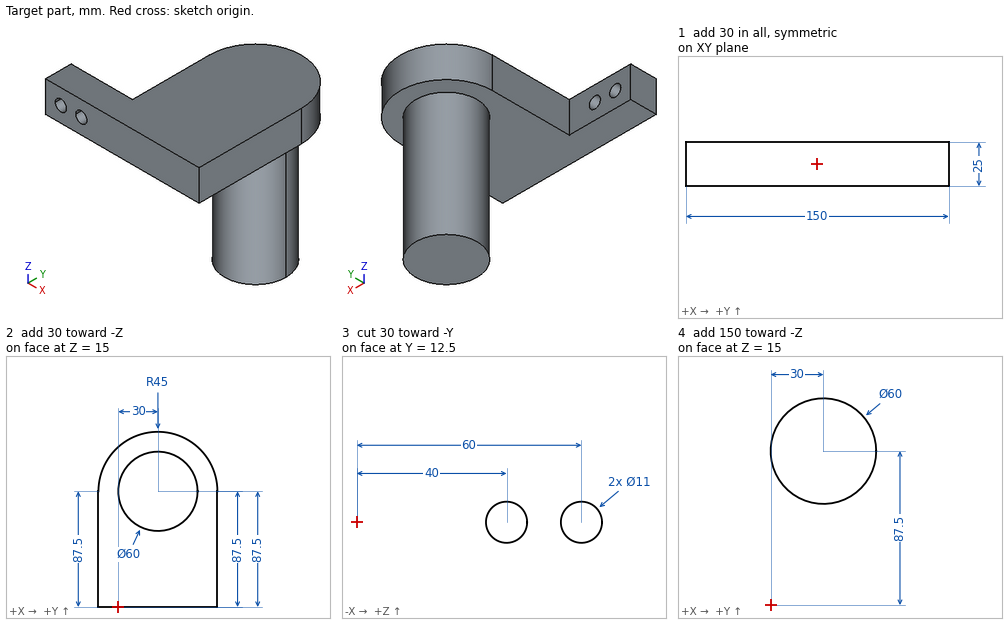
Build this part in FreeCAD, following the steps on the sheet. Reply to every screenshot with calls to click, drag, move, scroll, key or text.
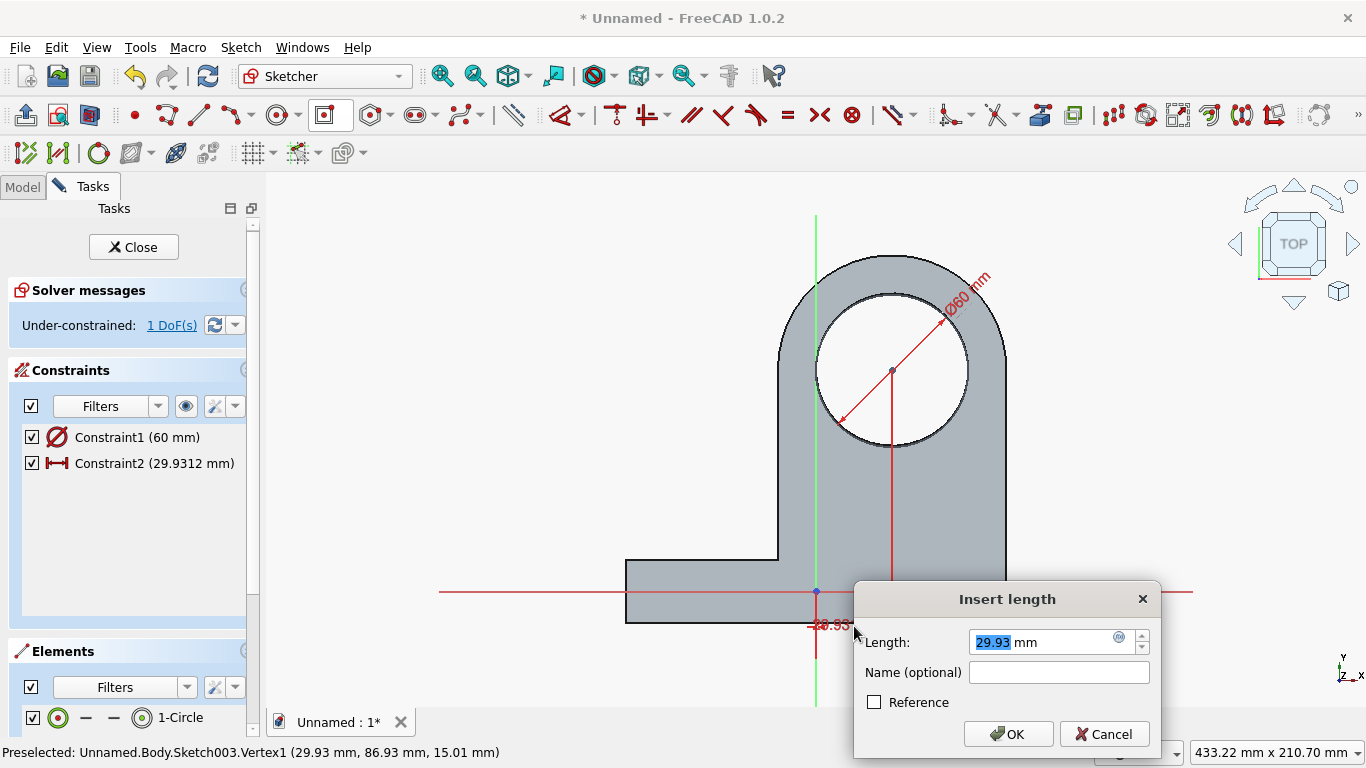
text(30)
key(Return)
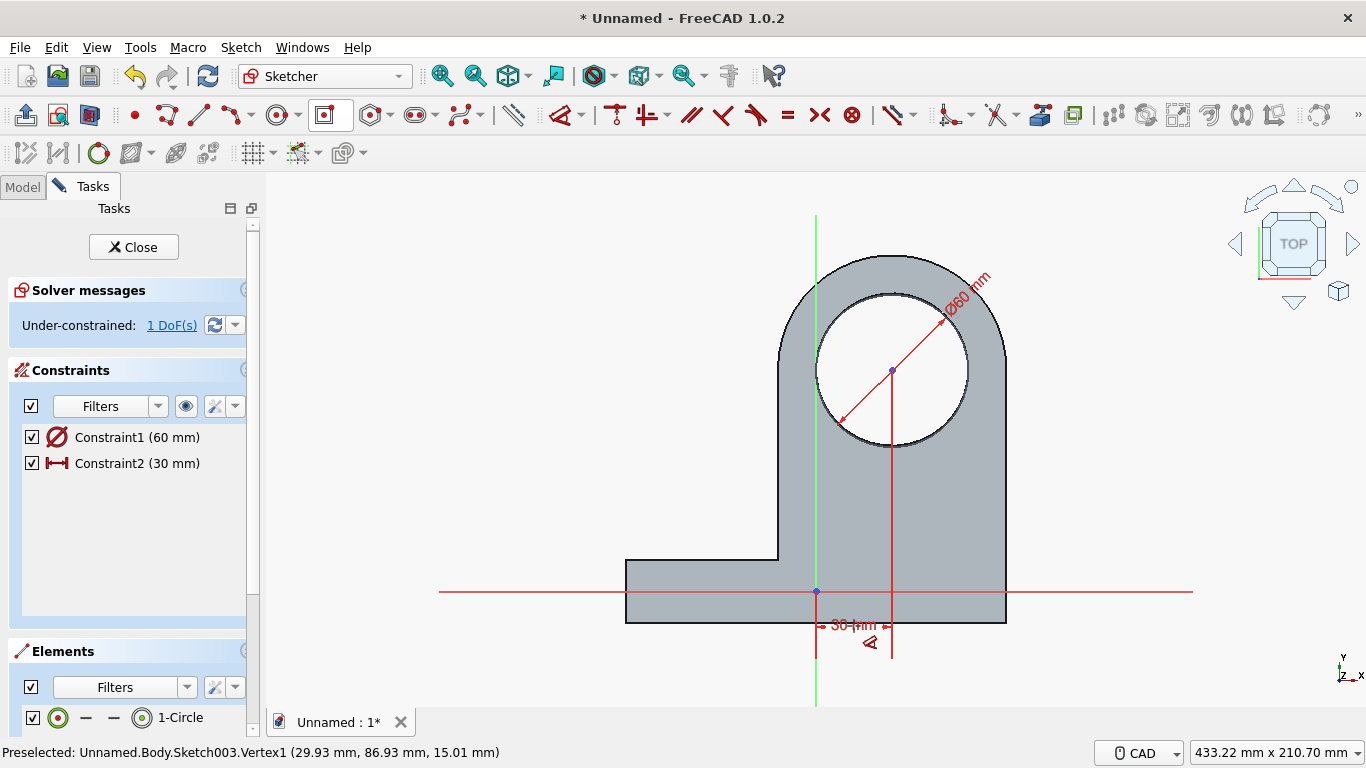
click(892, 371)
click(782, 481)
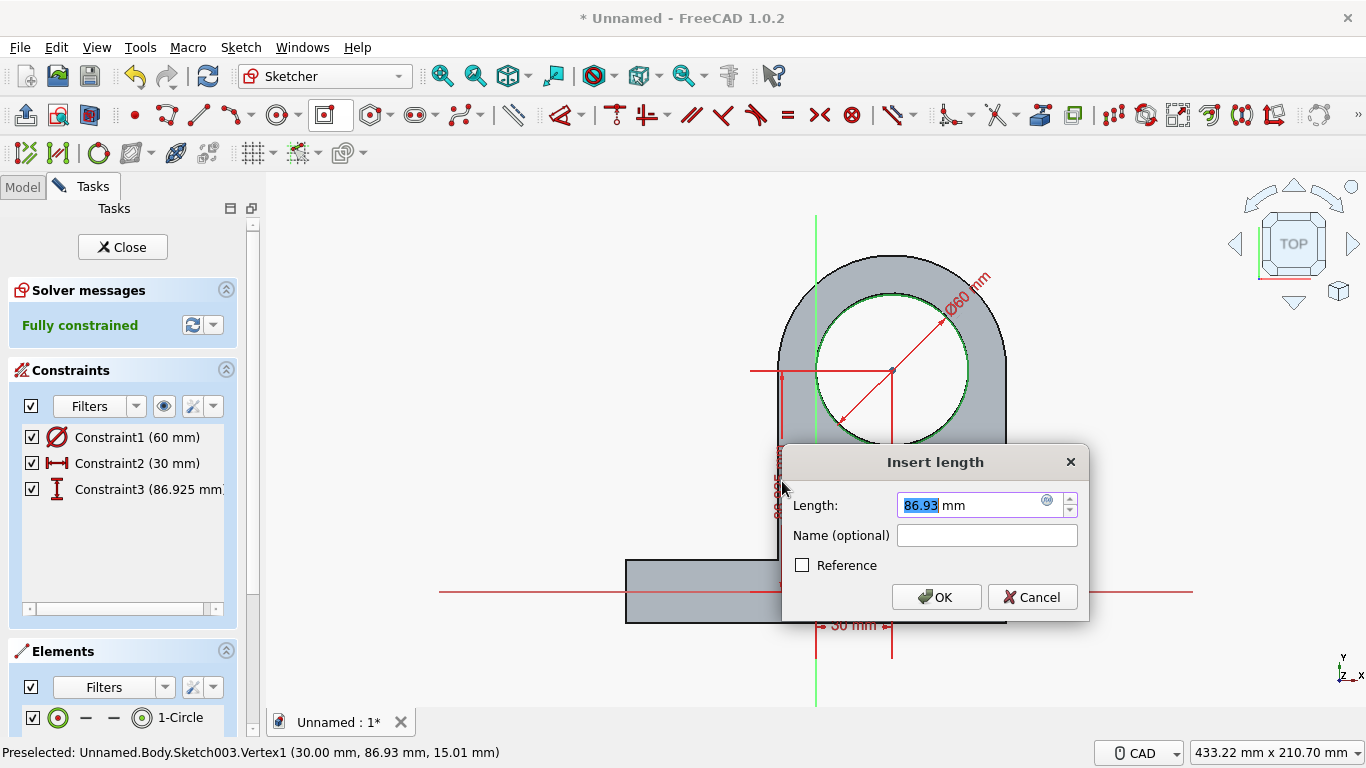
text(87.5)
key(Return)
key(Escape)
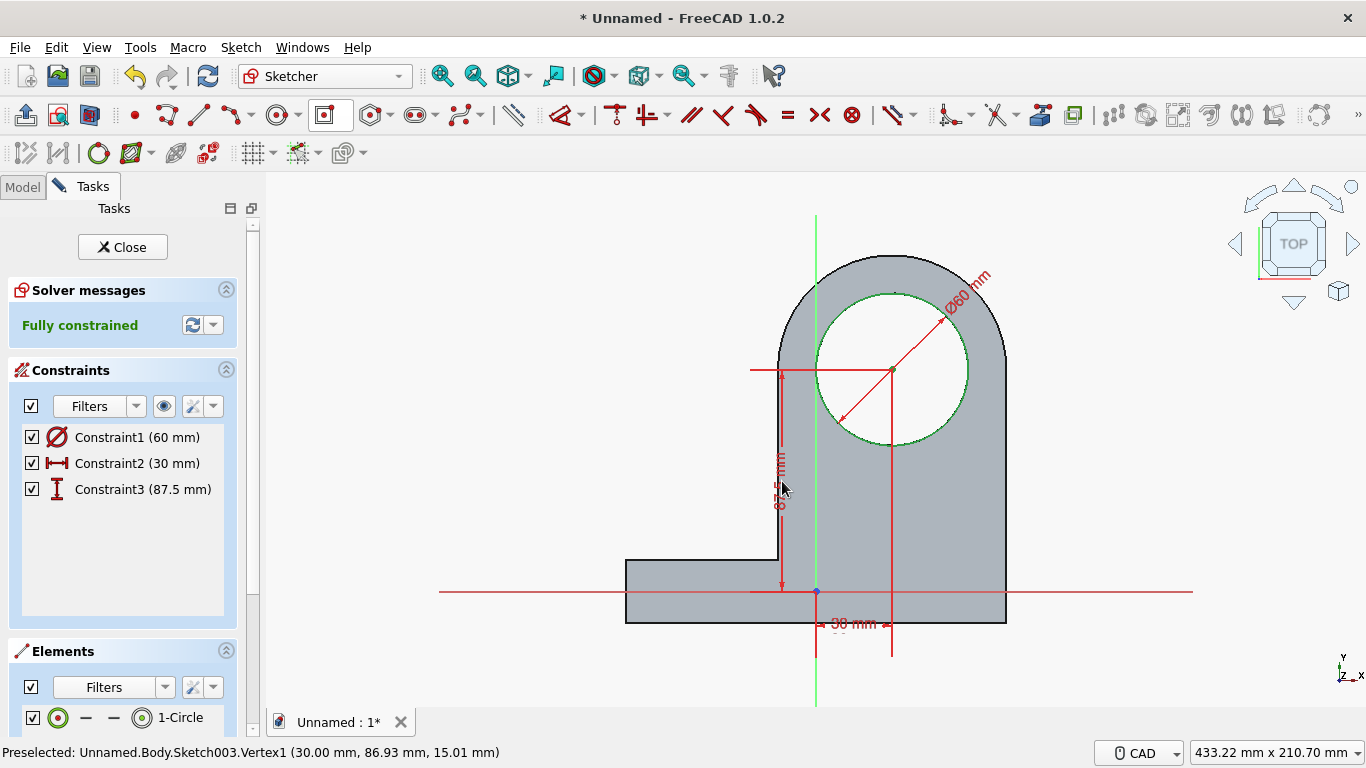
click(123, 247)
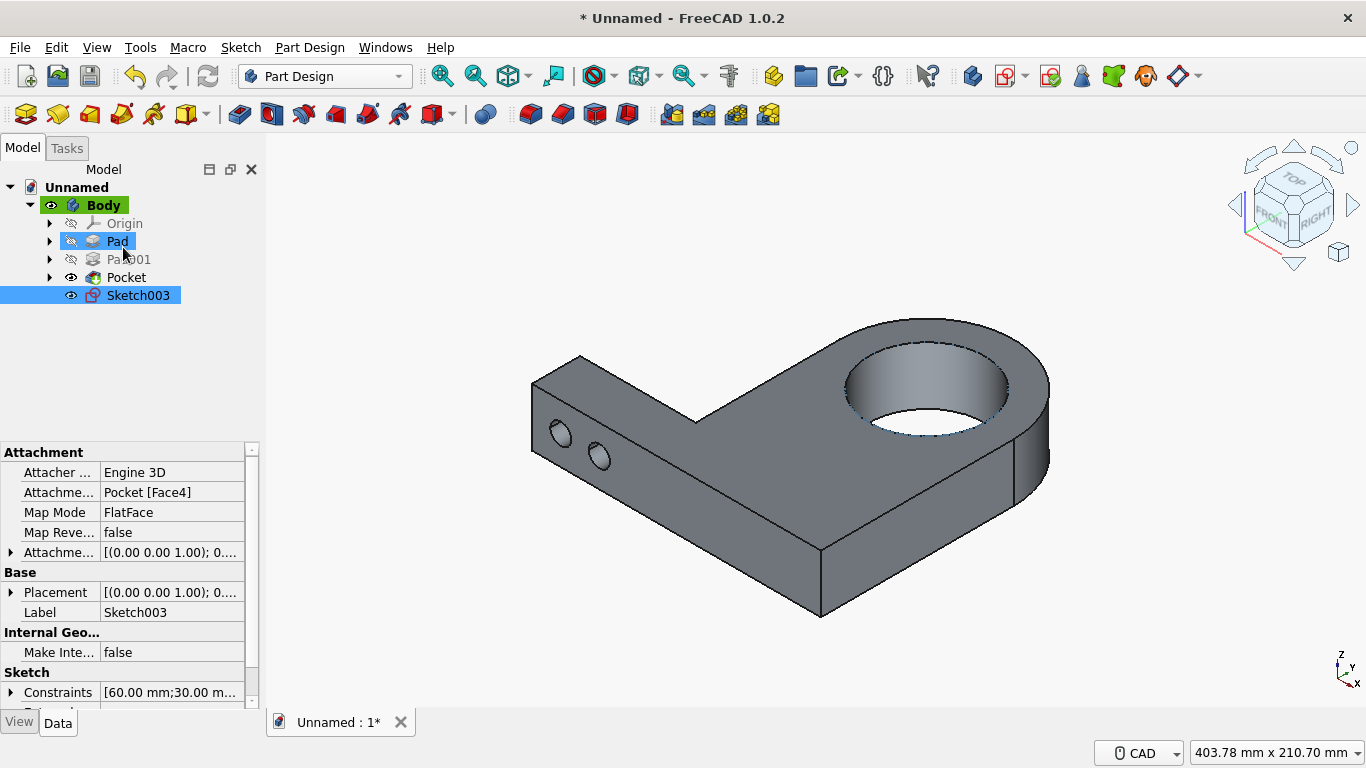
click(26, 114)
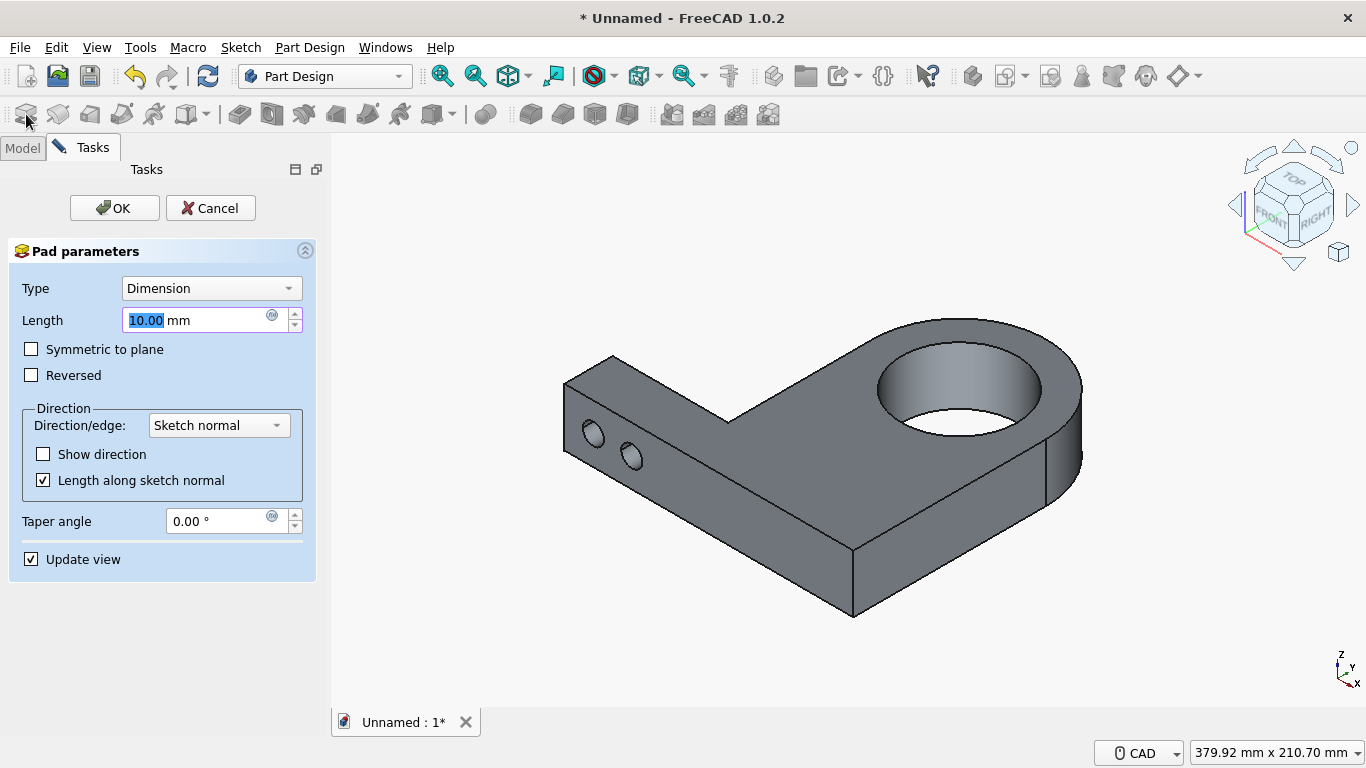
text(150)
key(Tab)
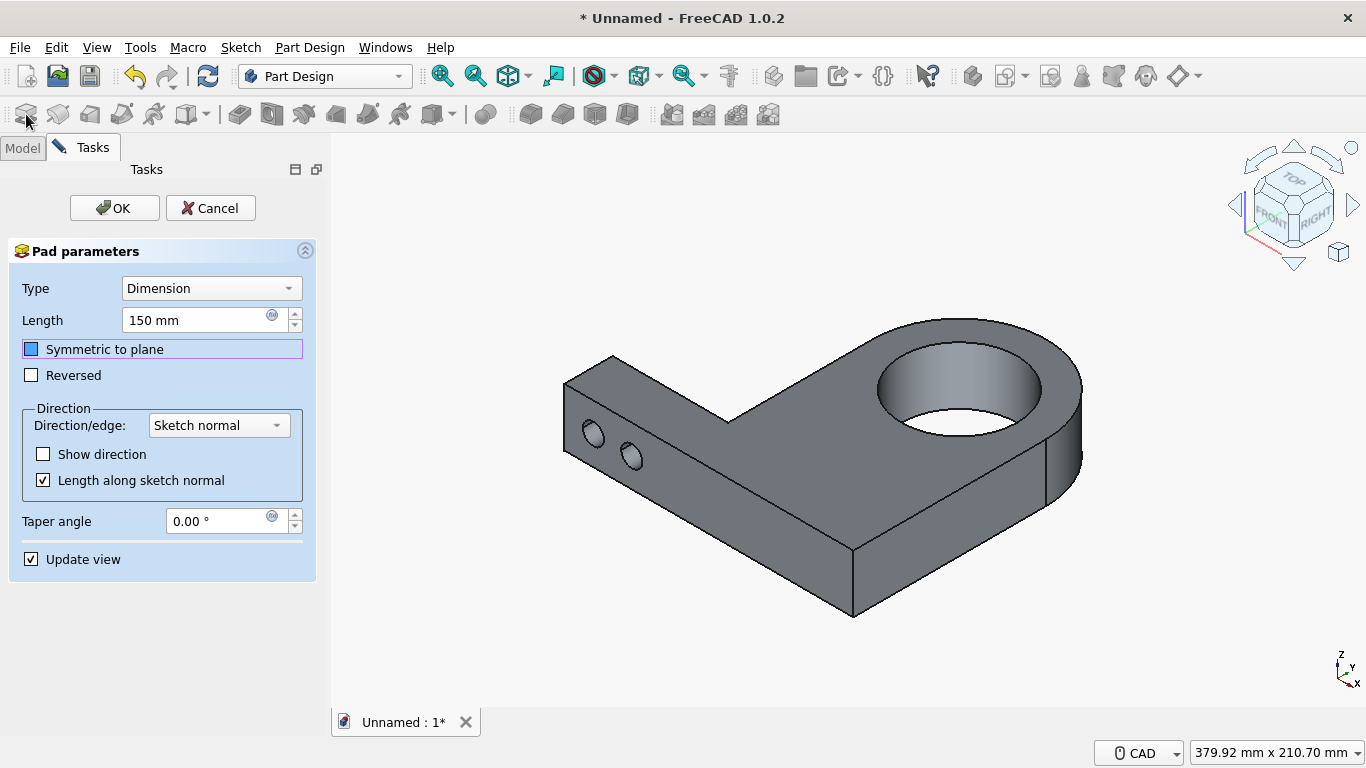
click(30, 375)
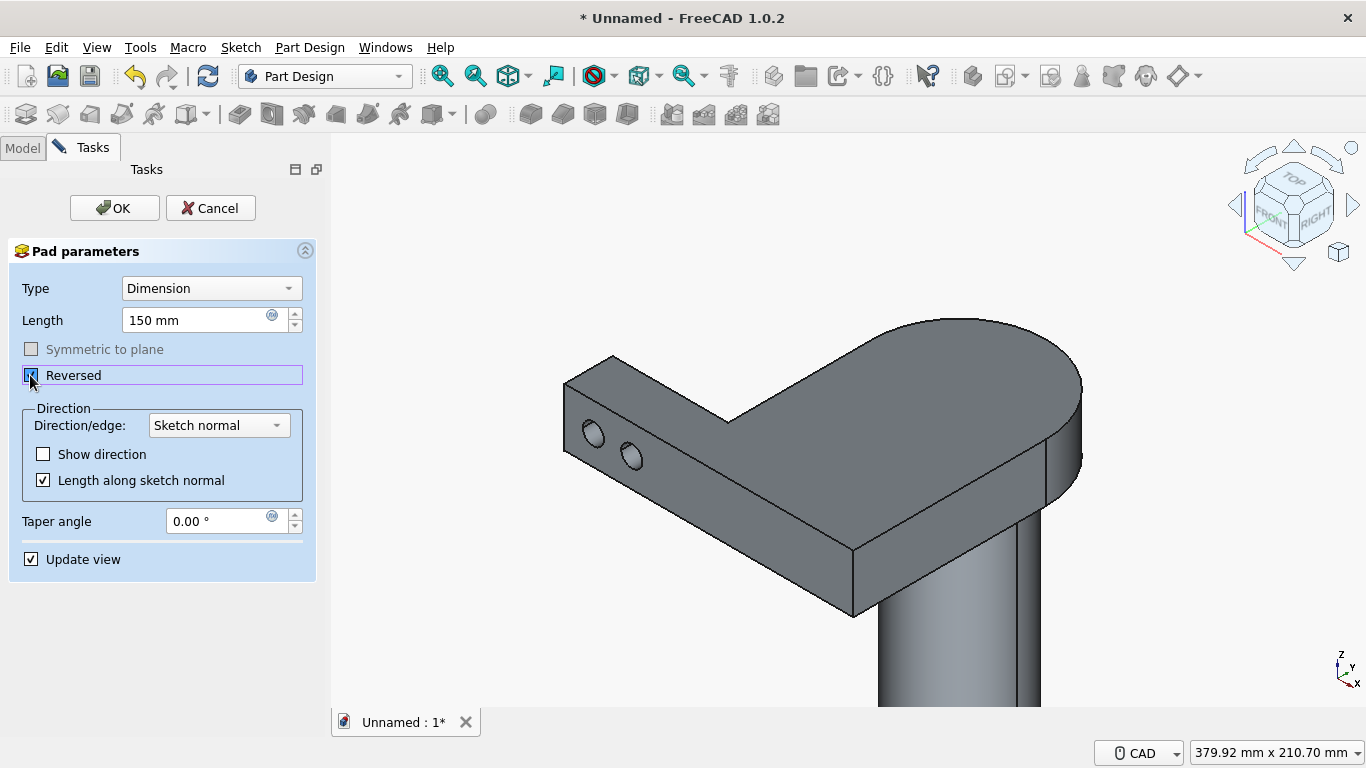
click(115, 208)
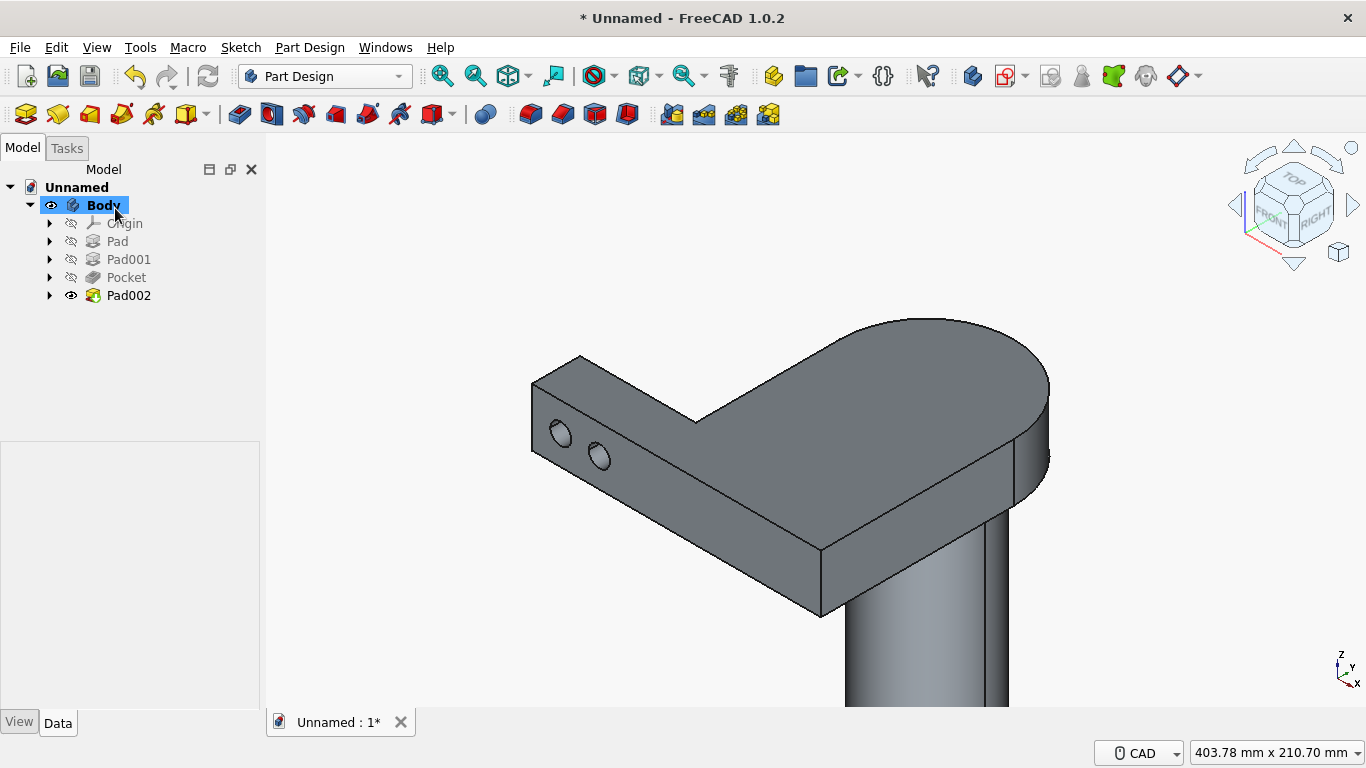
click(444, 76)